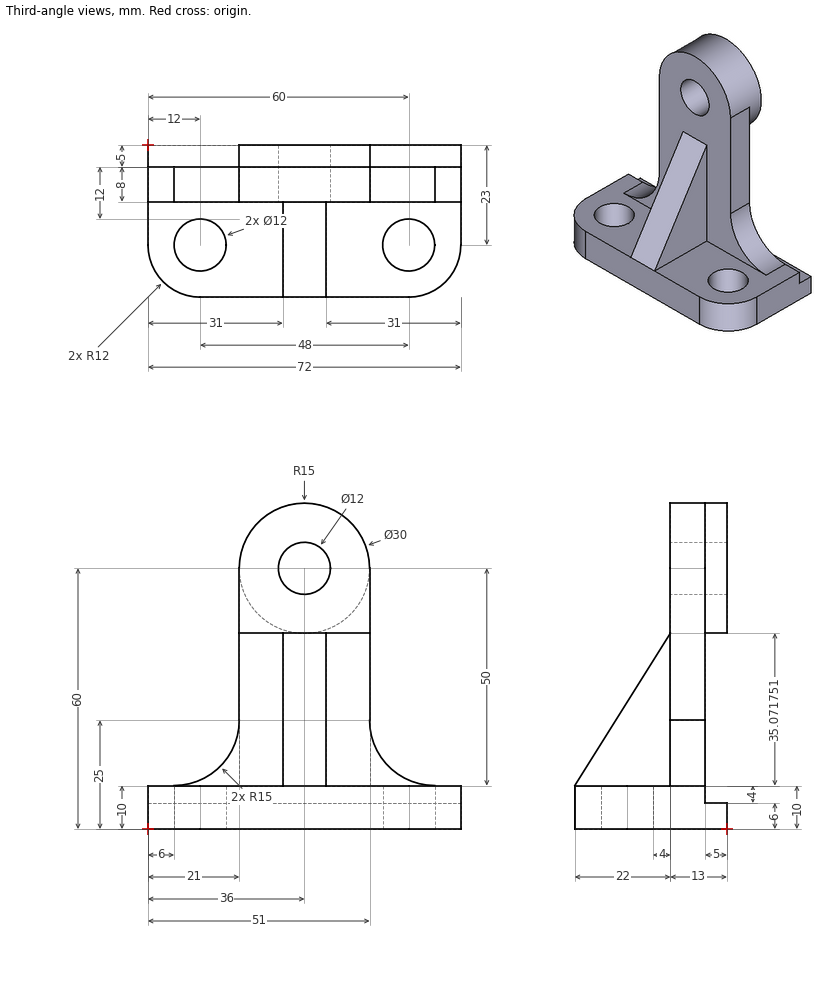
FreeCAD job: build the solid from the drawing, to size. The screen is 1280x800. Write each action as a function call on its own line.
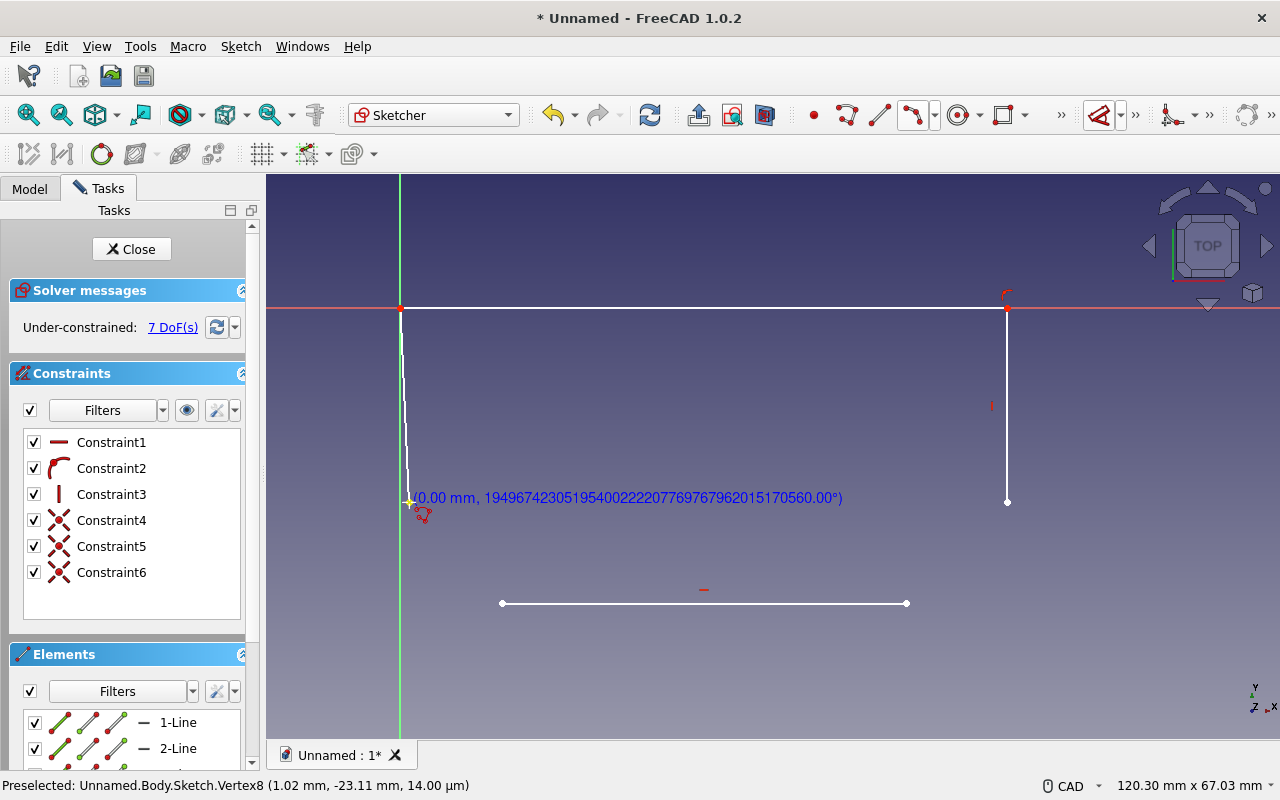
click(912, 116)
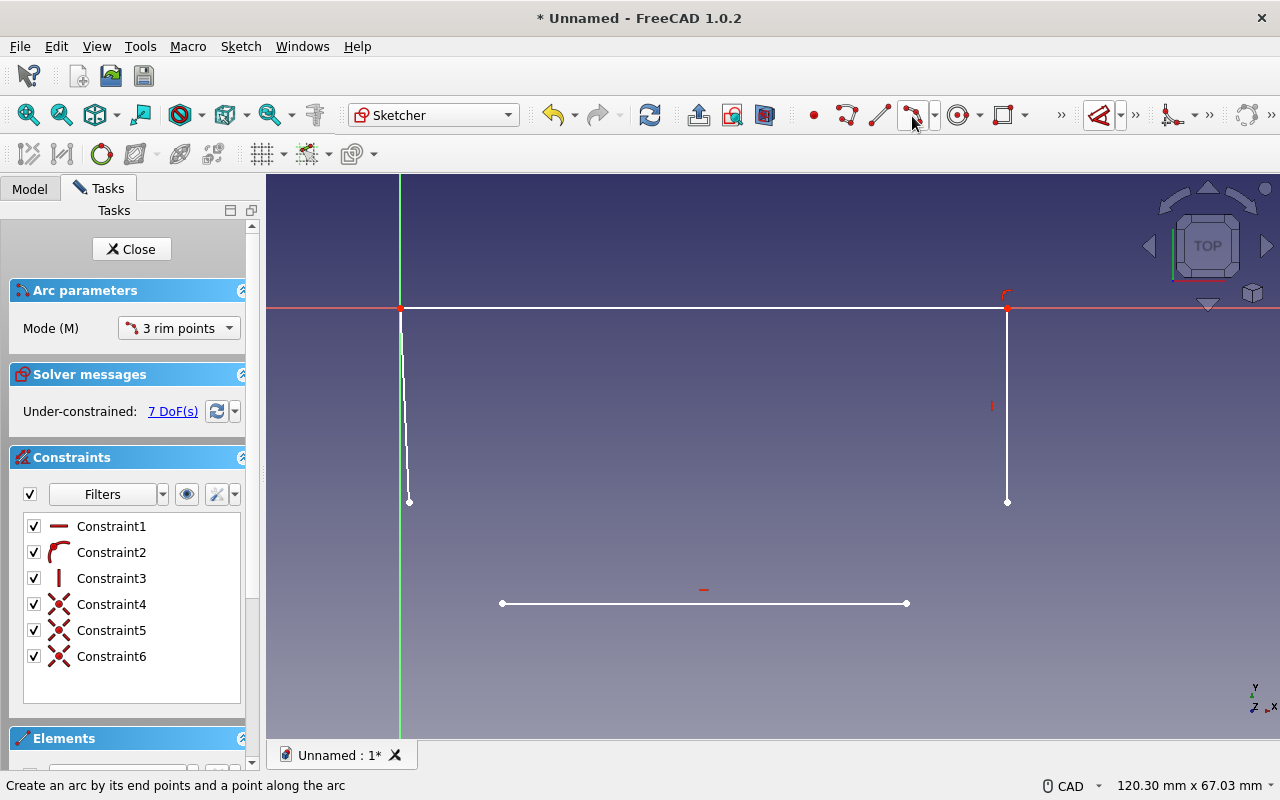
click(906, 604)
click(1007, 503)
click(978, 574)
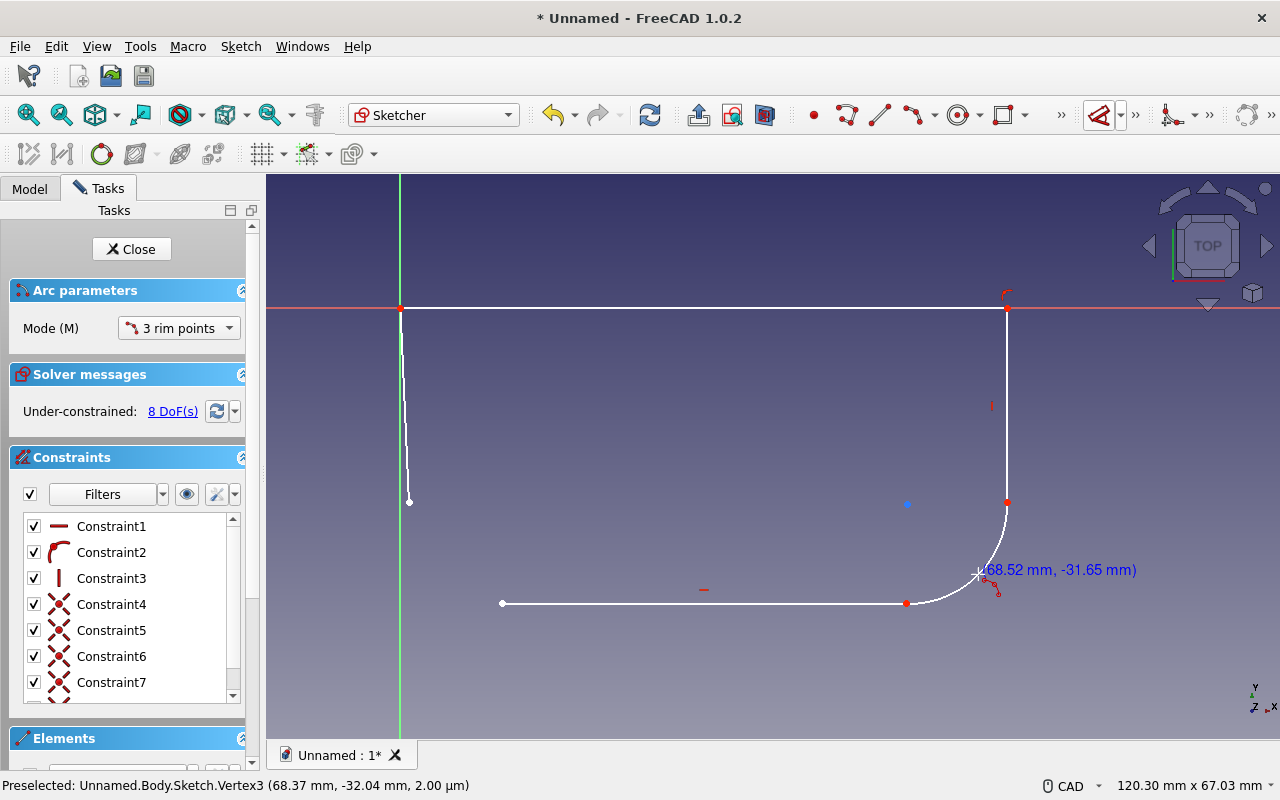
click(409, 503)
click(502, 604)
click(430, 574)
key(Escape)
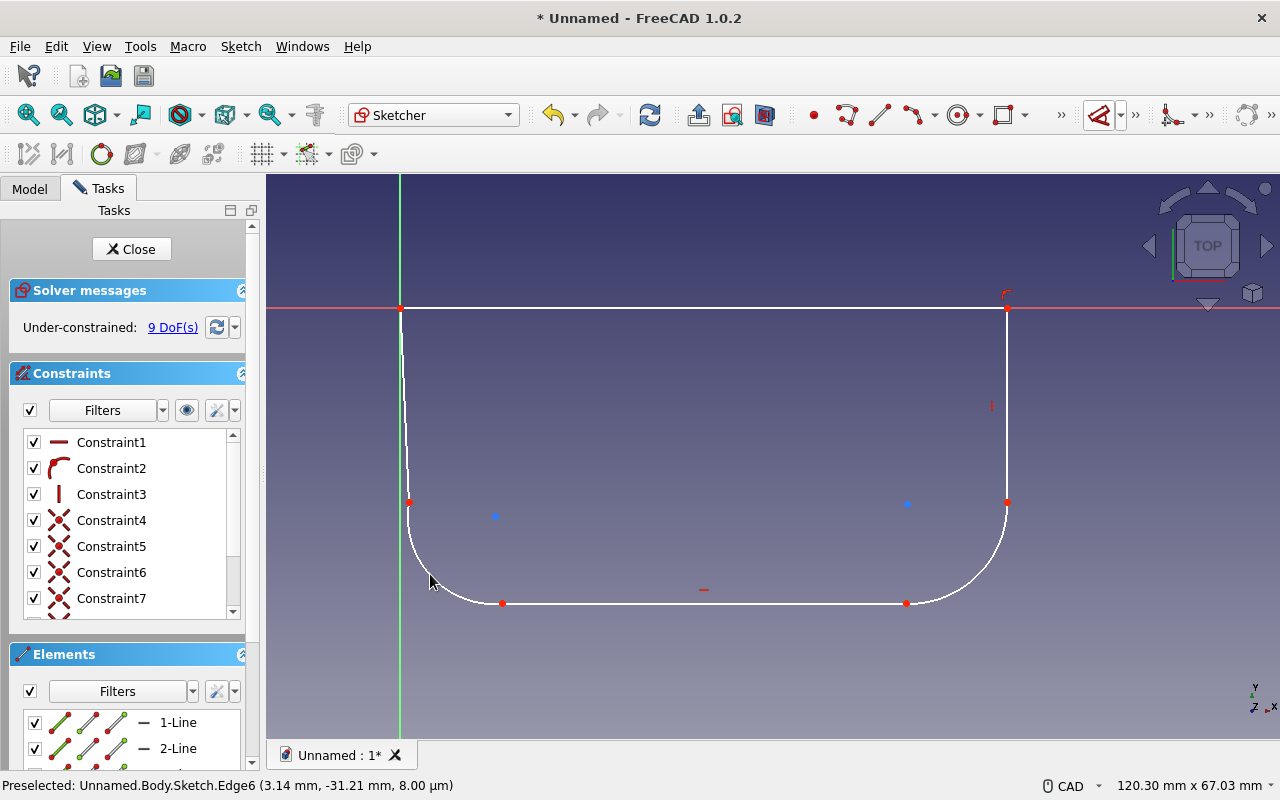
click(623, 604)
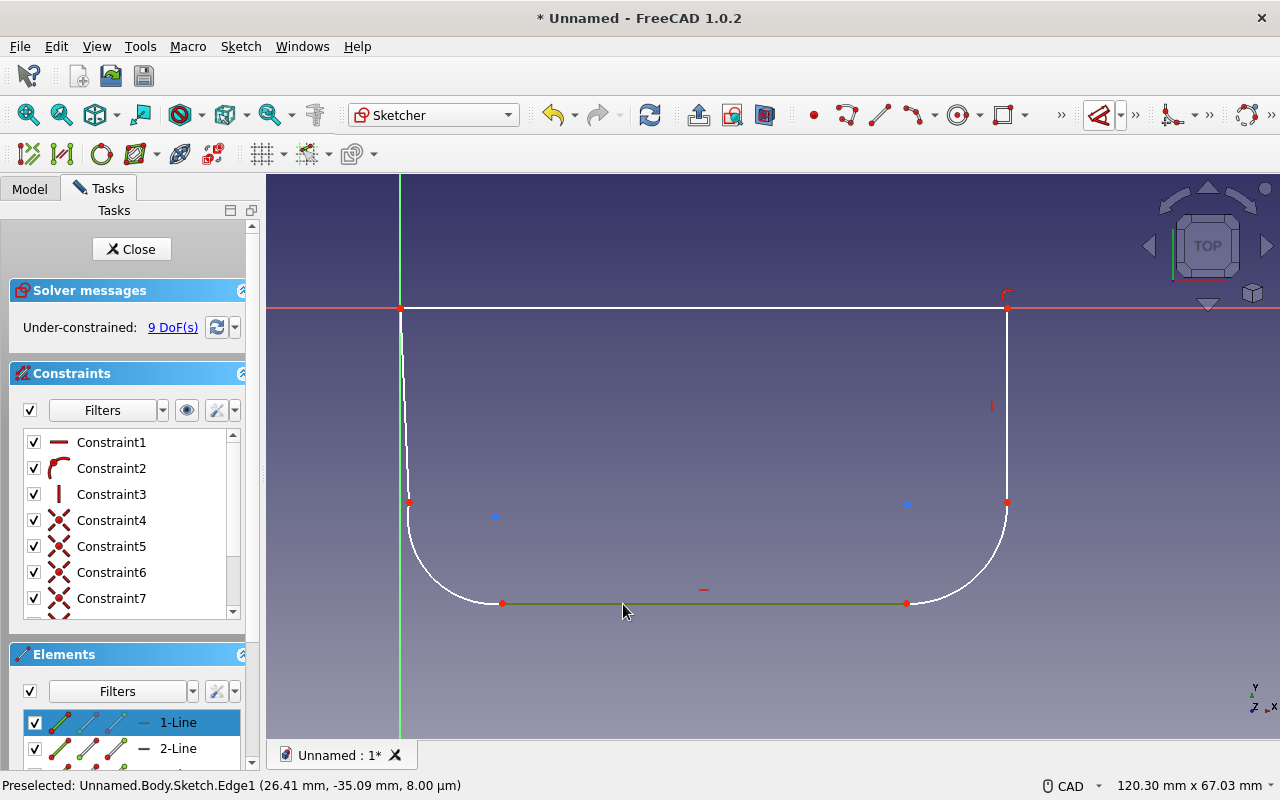
click(952, 594)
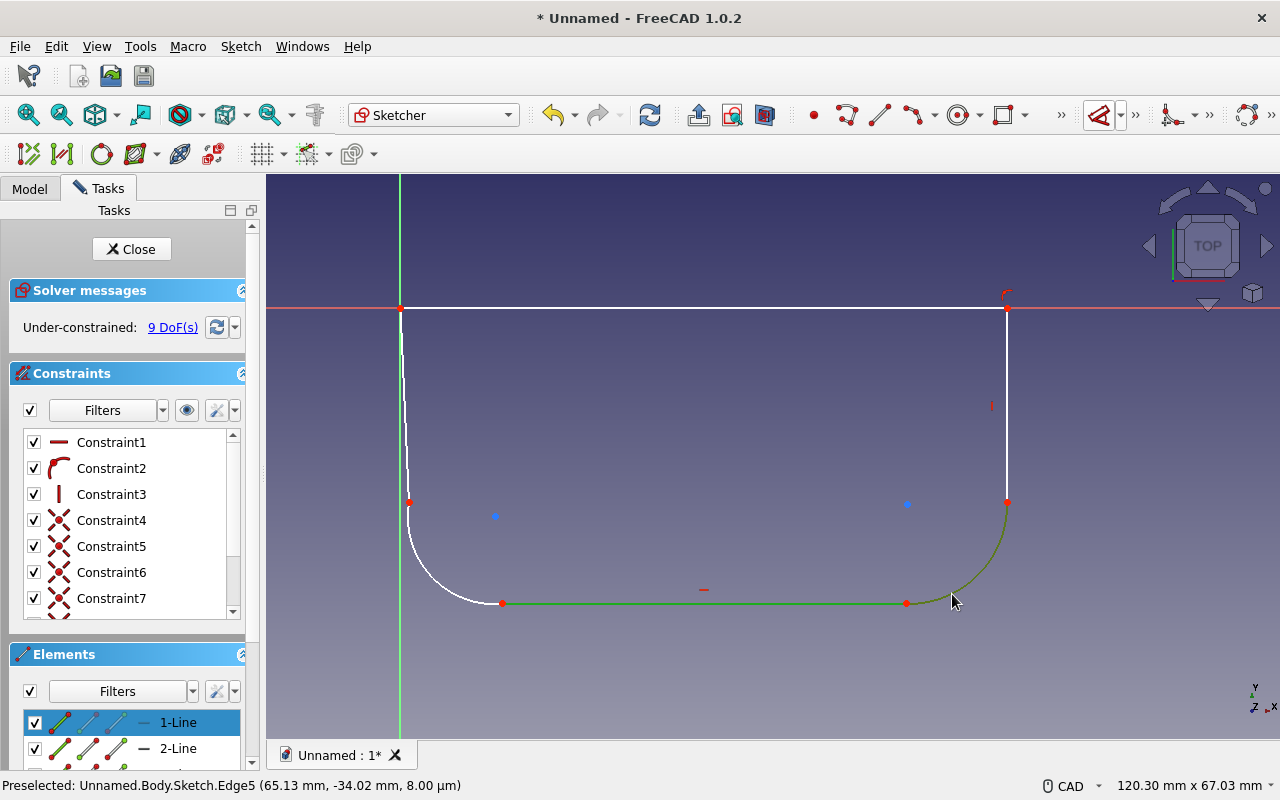
key(t)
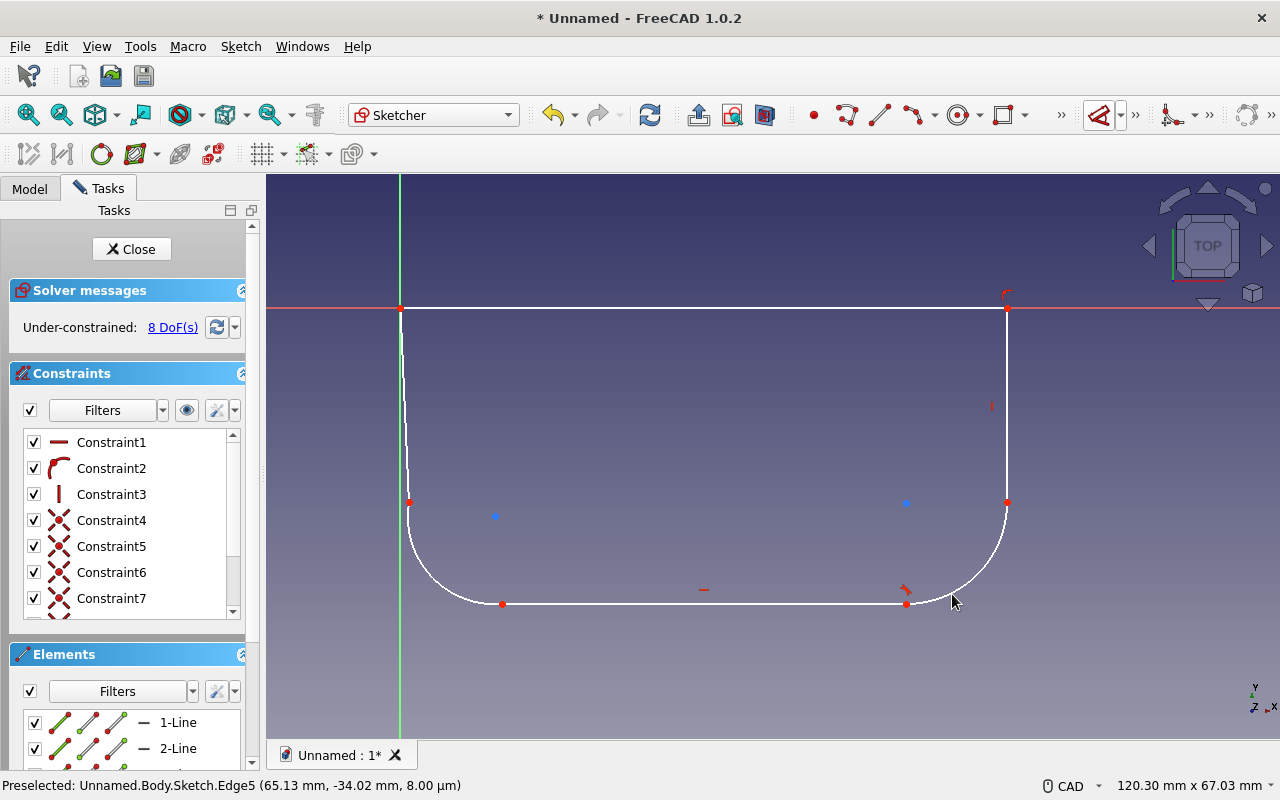
click(623, 604)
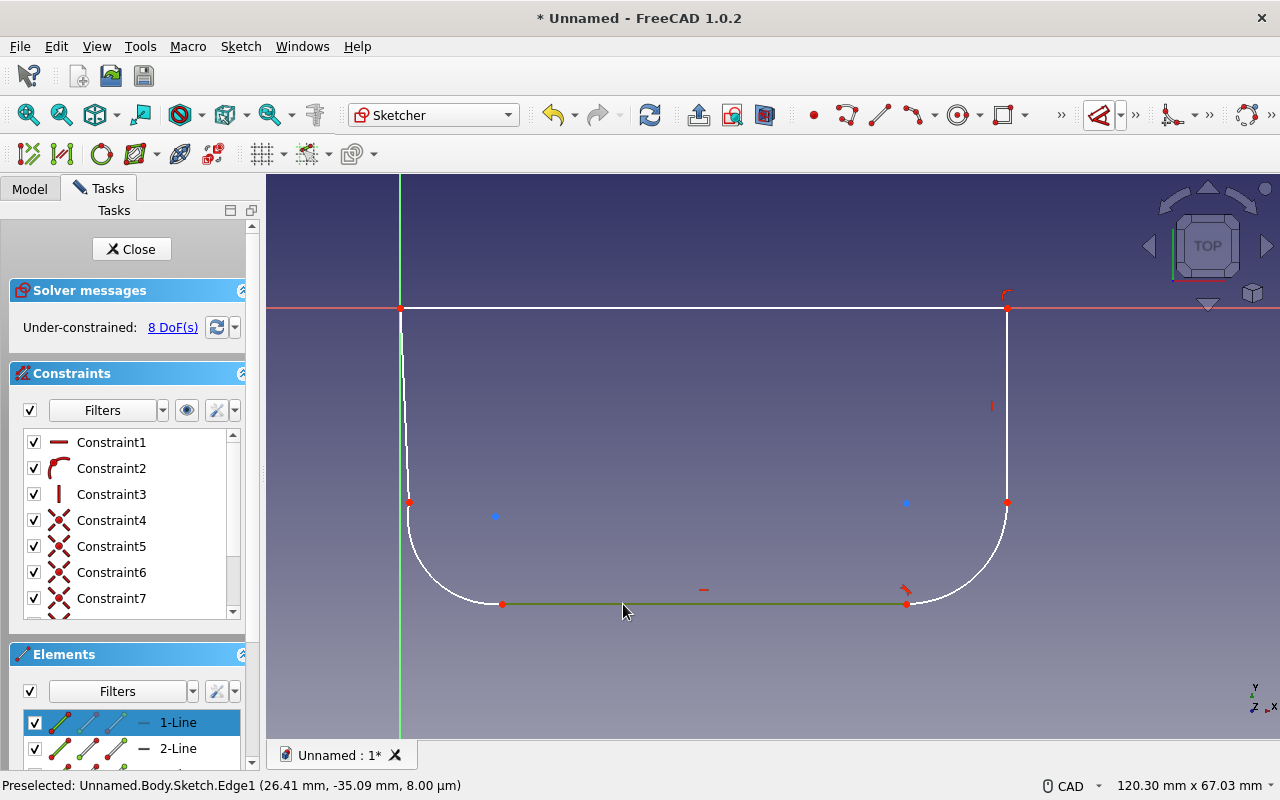
click(414, 550)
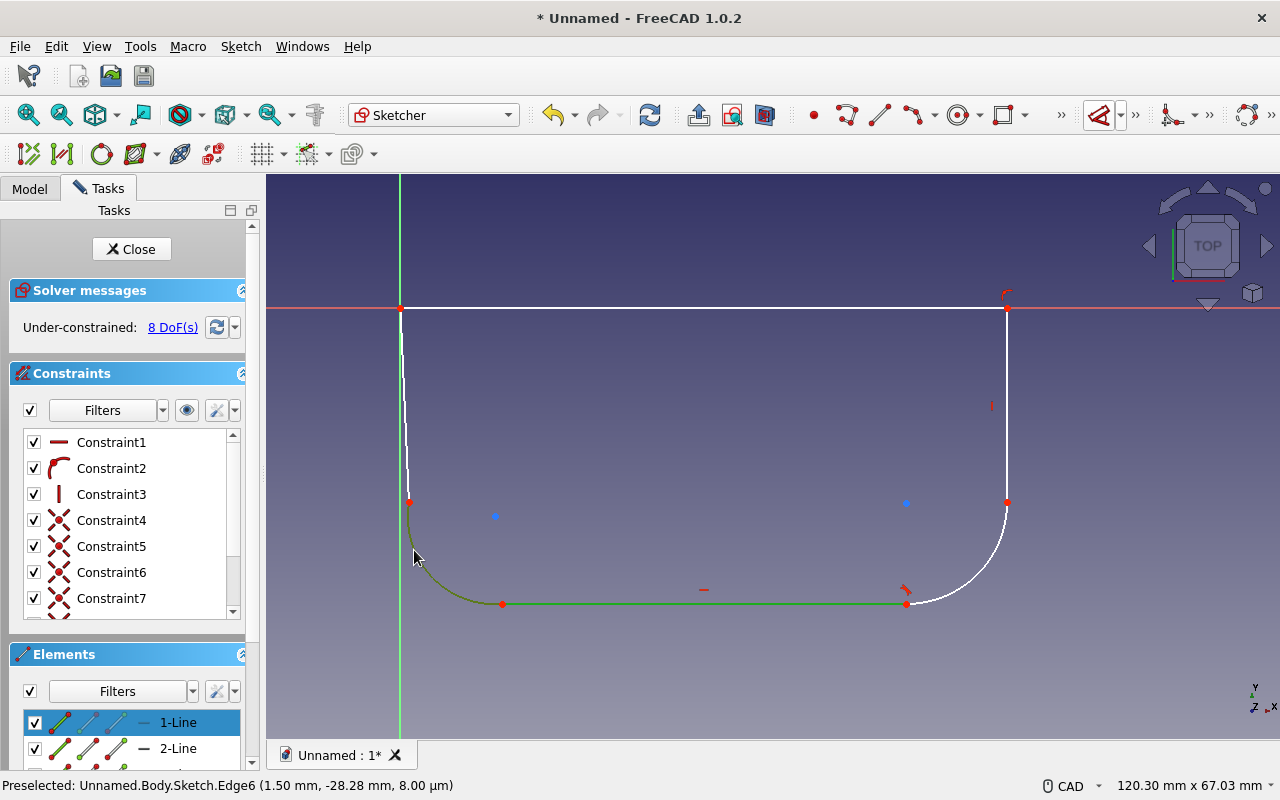
key(t)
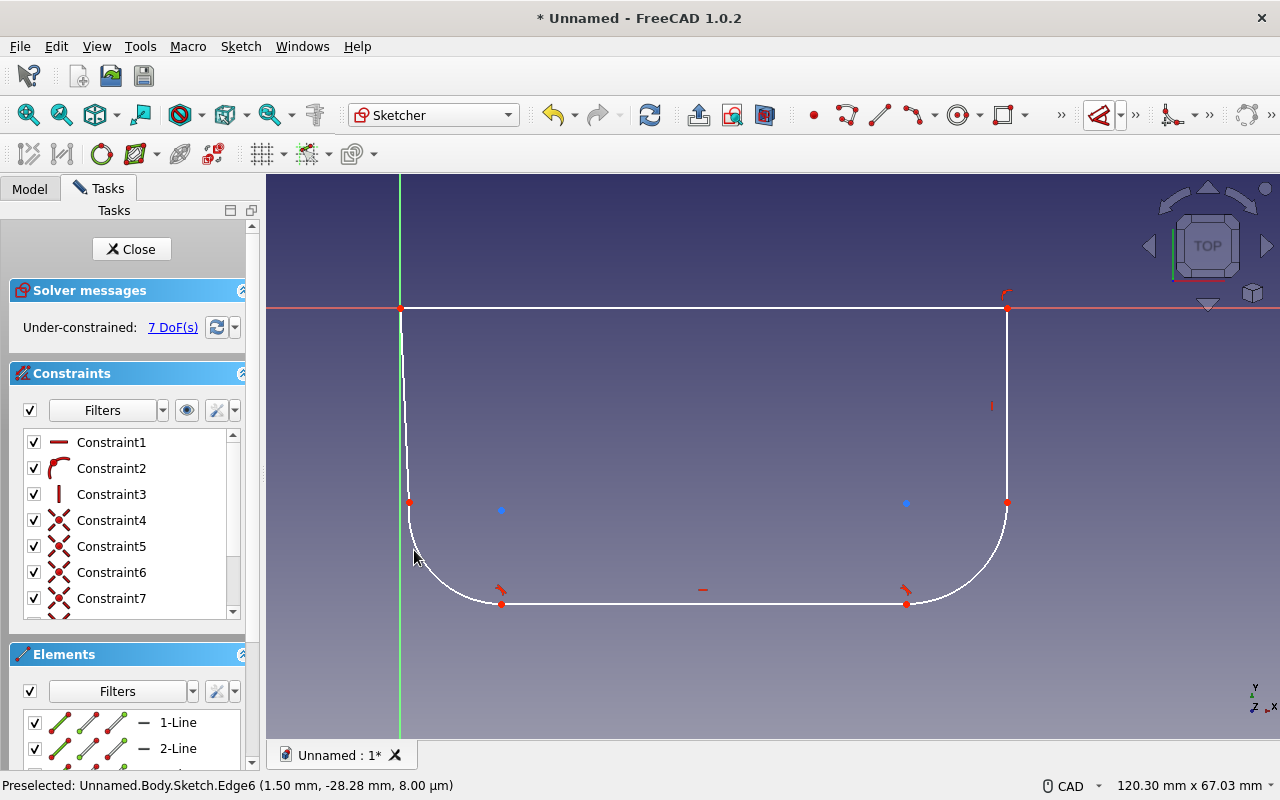
click(1007, 445)